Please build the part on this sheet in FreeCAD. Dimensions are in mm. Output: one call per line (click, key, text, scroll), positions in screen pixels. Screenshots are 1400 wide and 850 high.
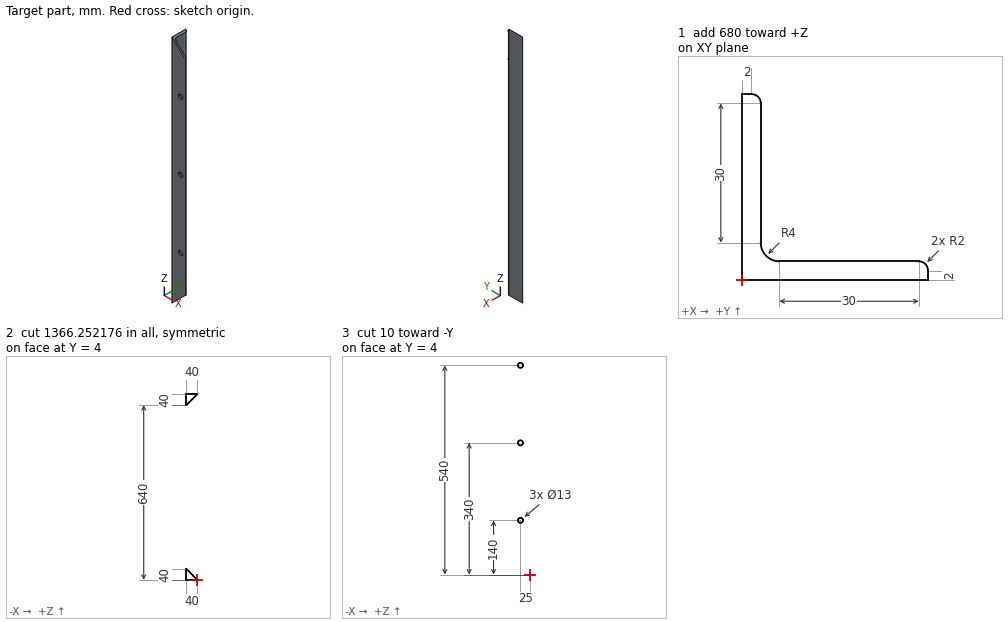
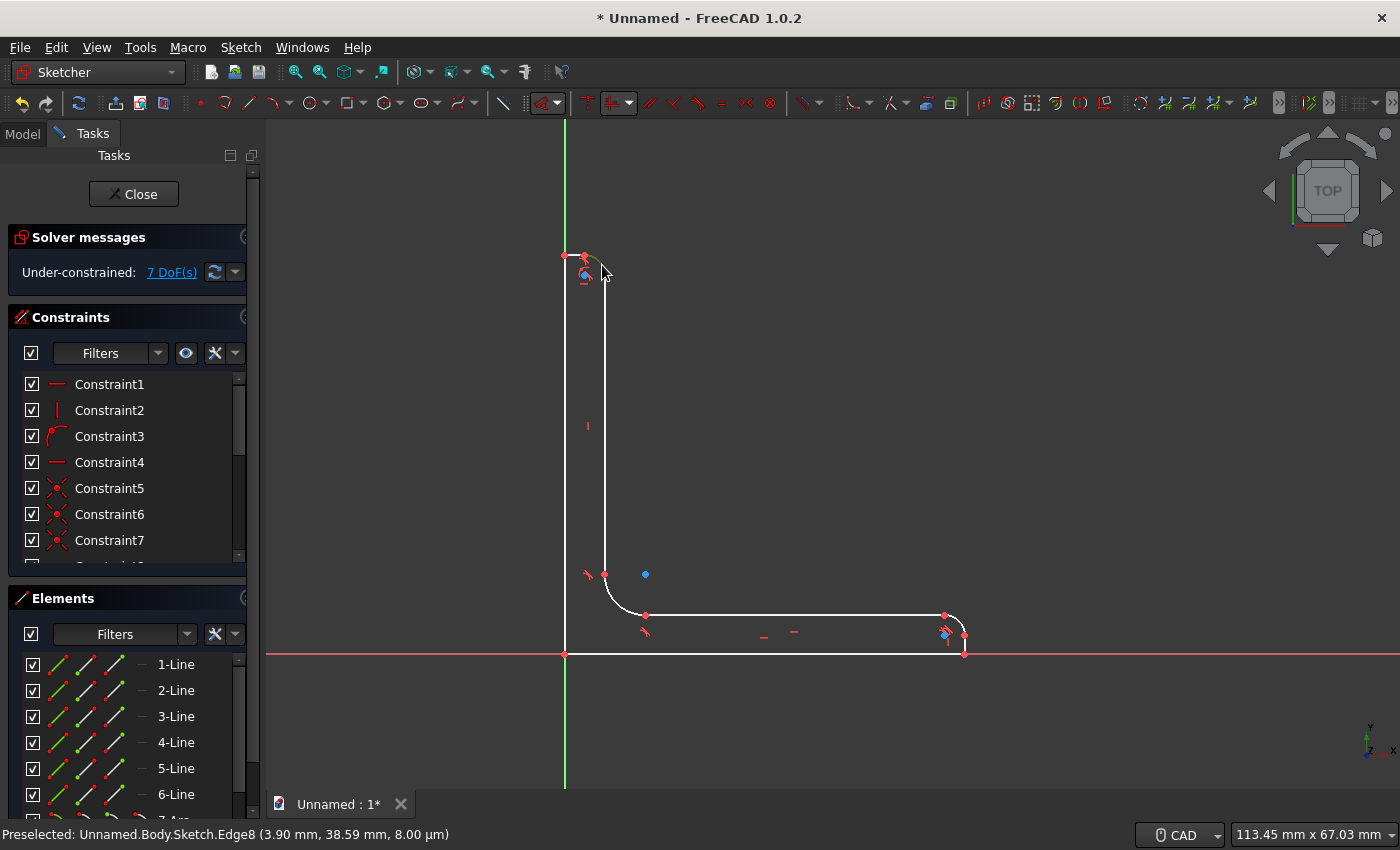
scroll(963, 626, up, 2)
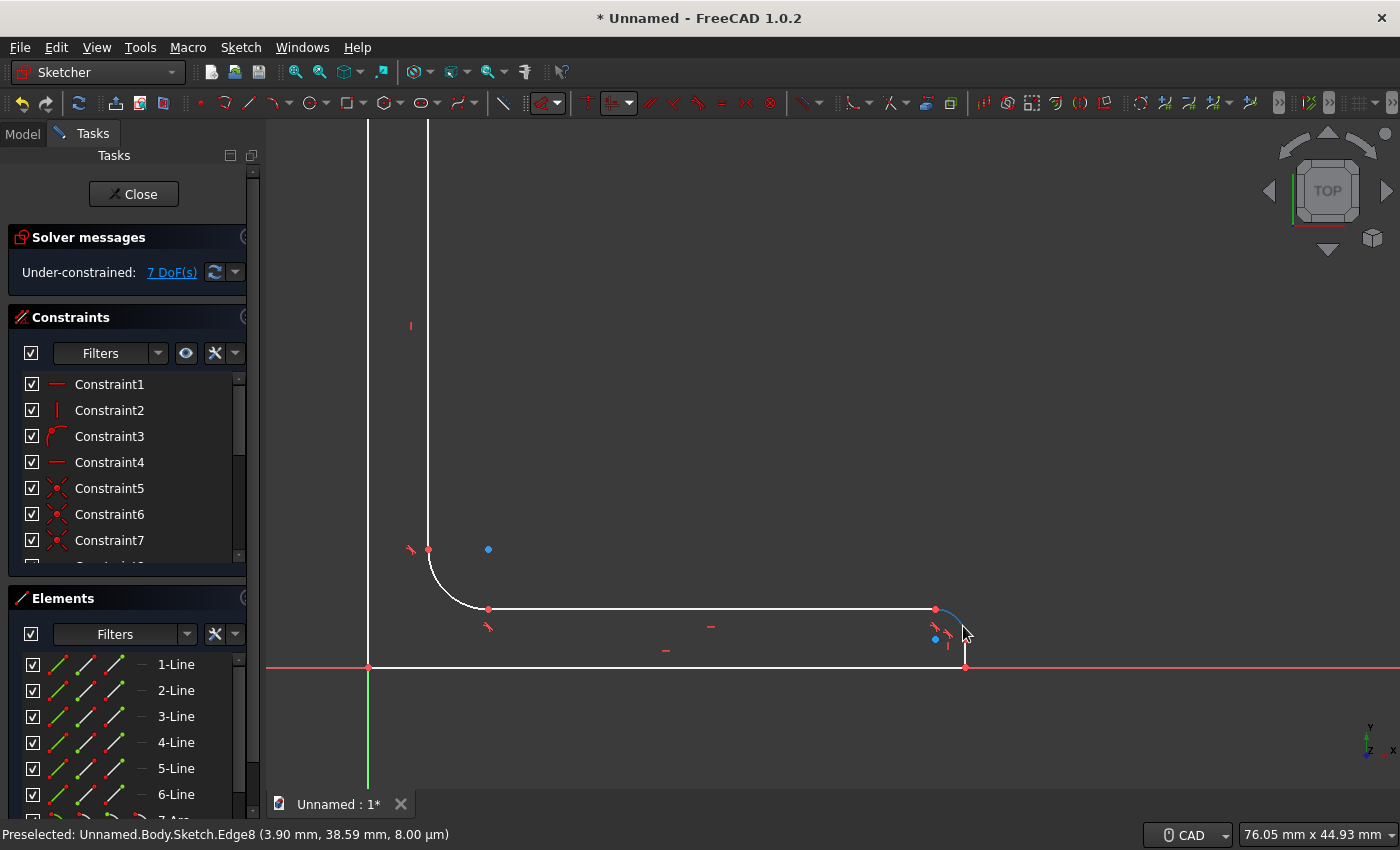
click(962, 626)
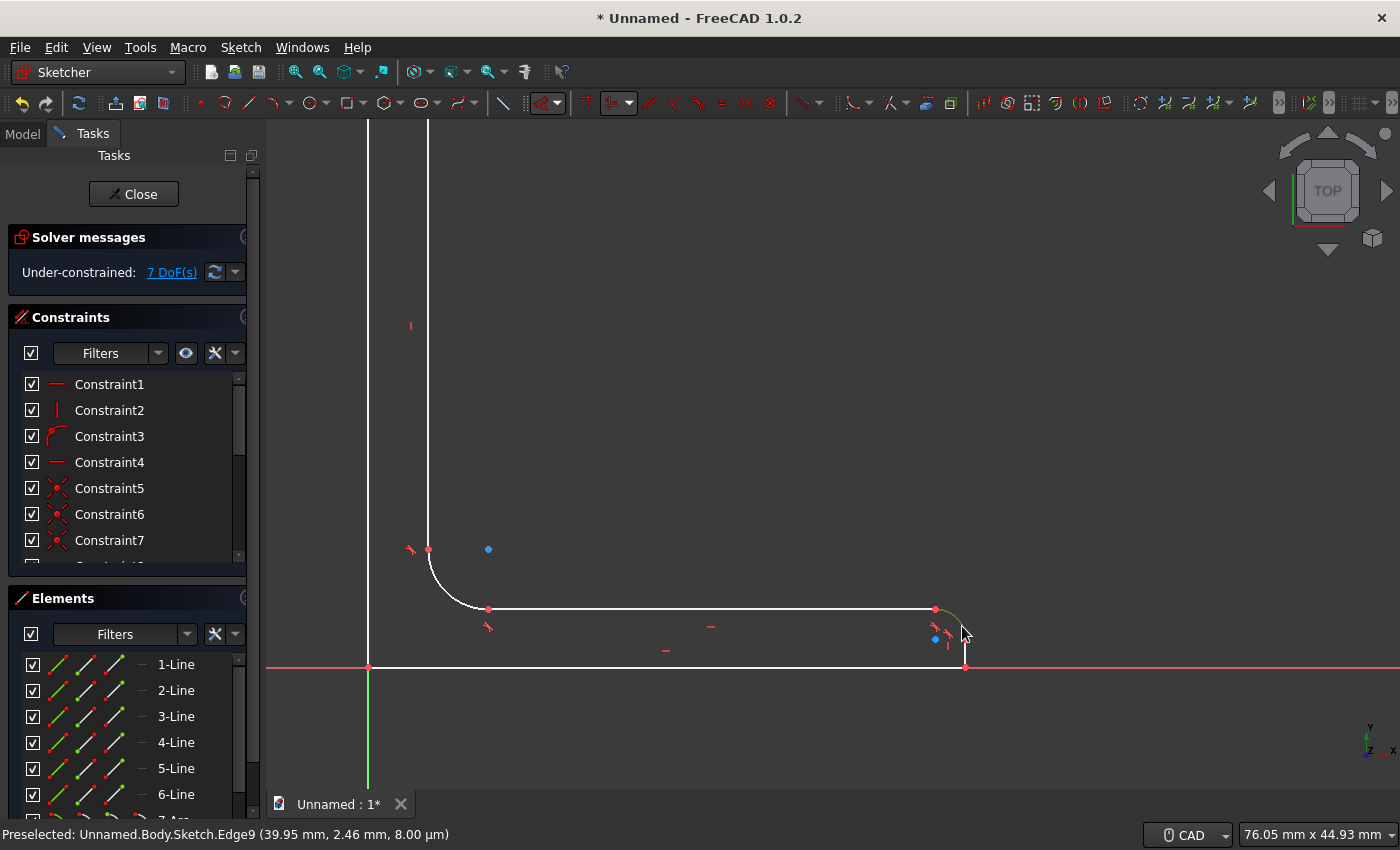
click(722, 104)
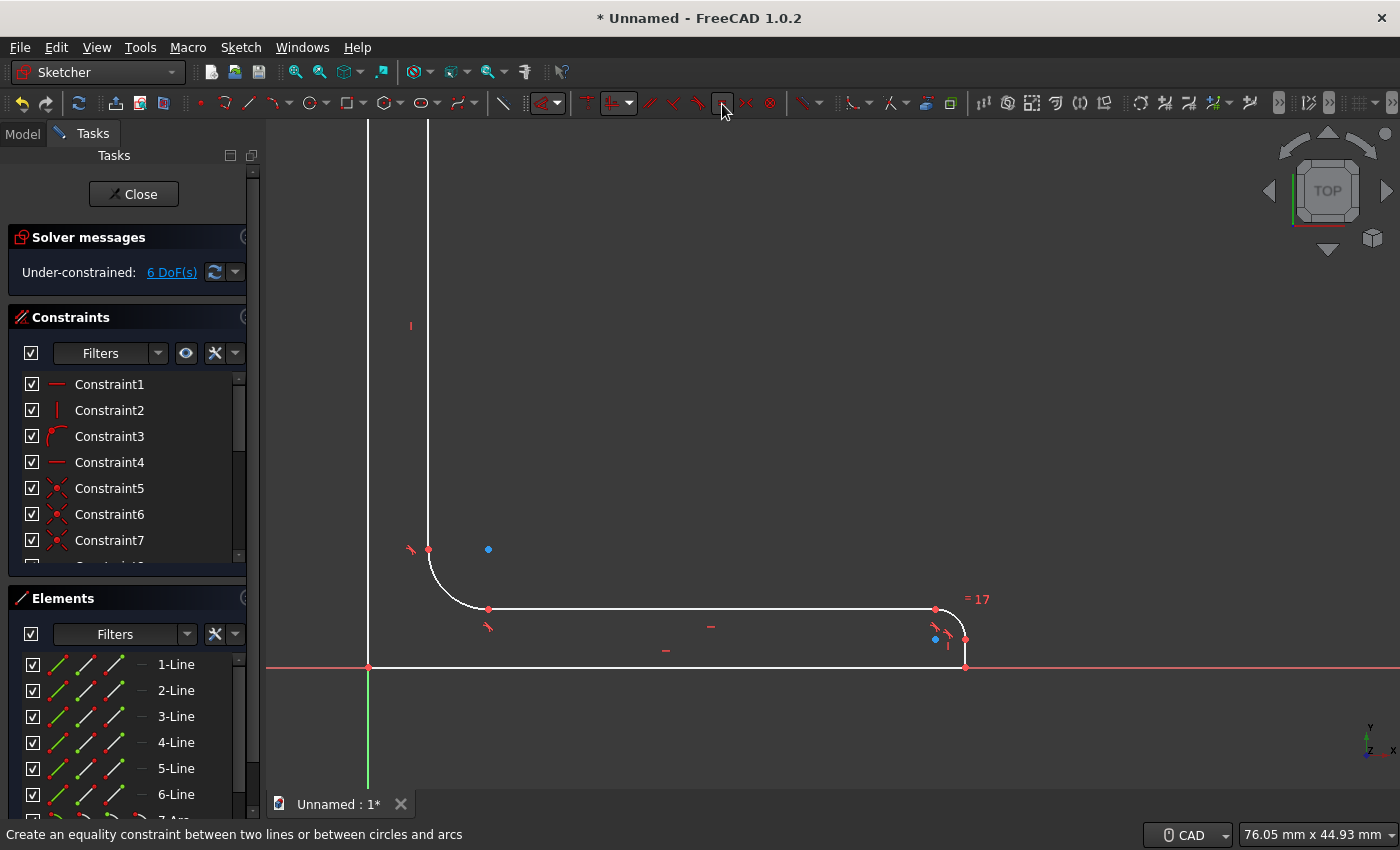
click(435, 577)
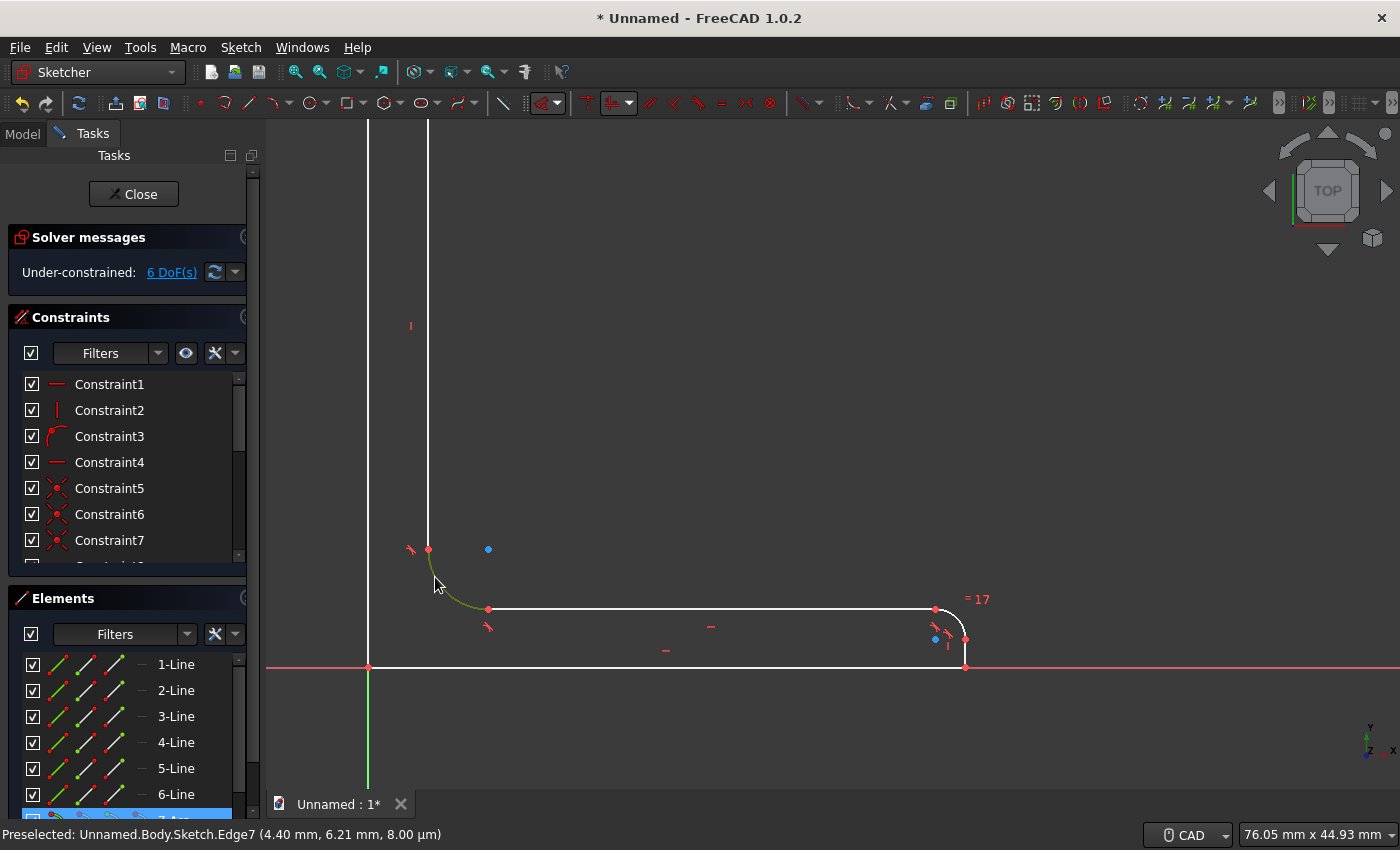
click(560, 104)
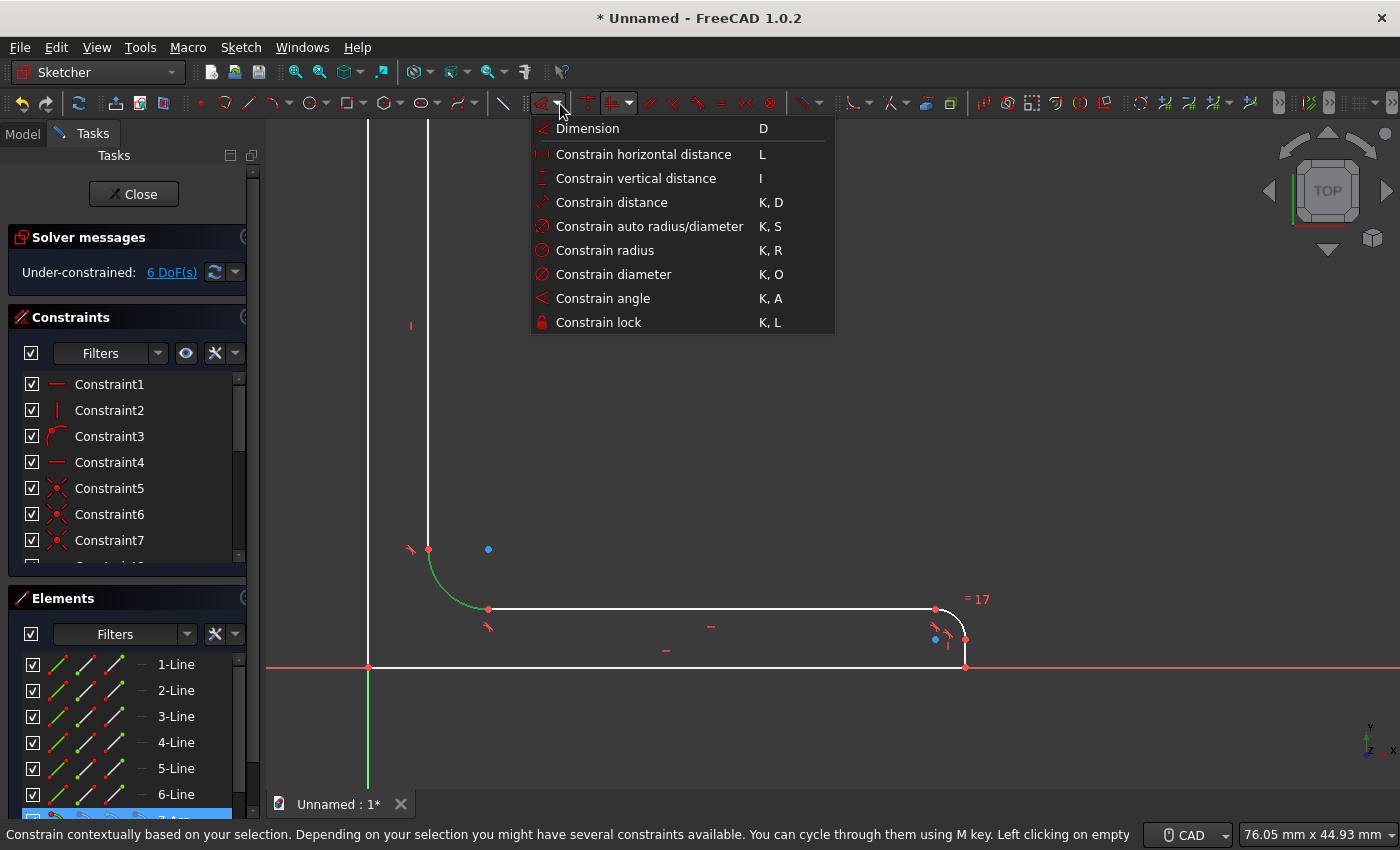
click(683, 250)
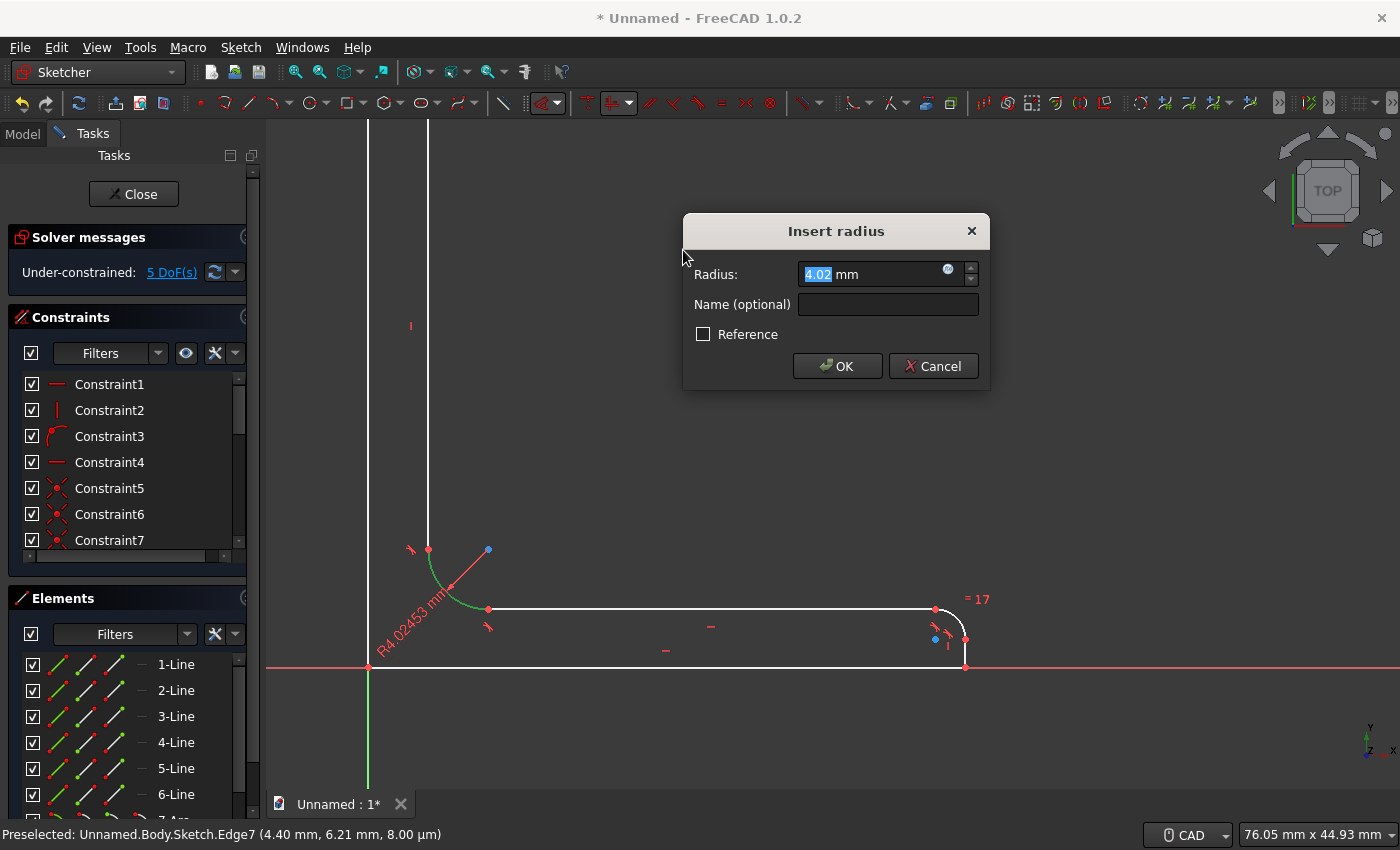
text(4)
key(Return)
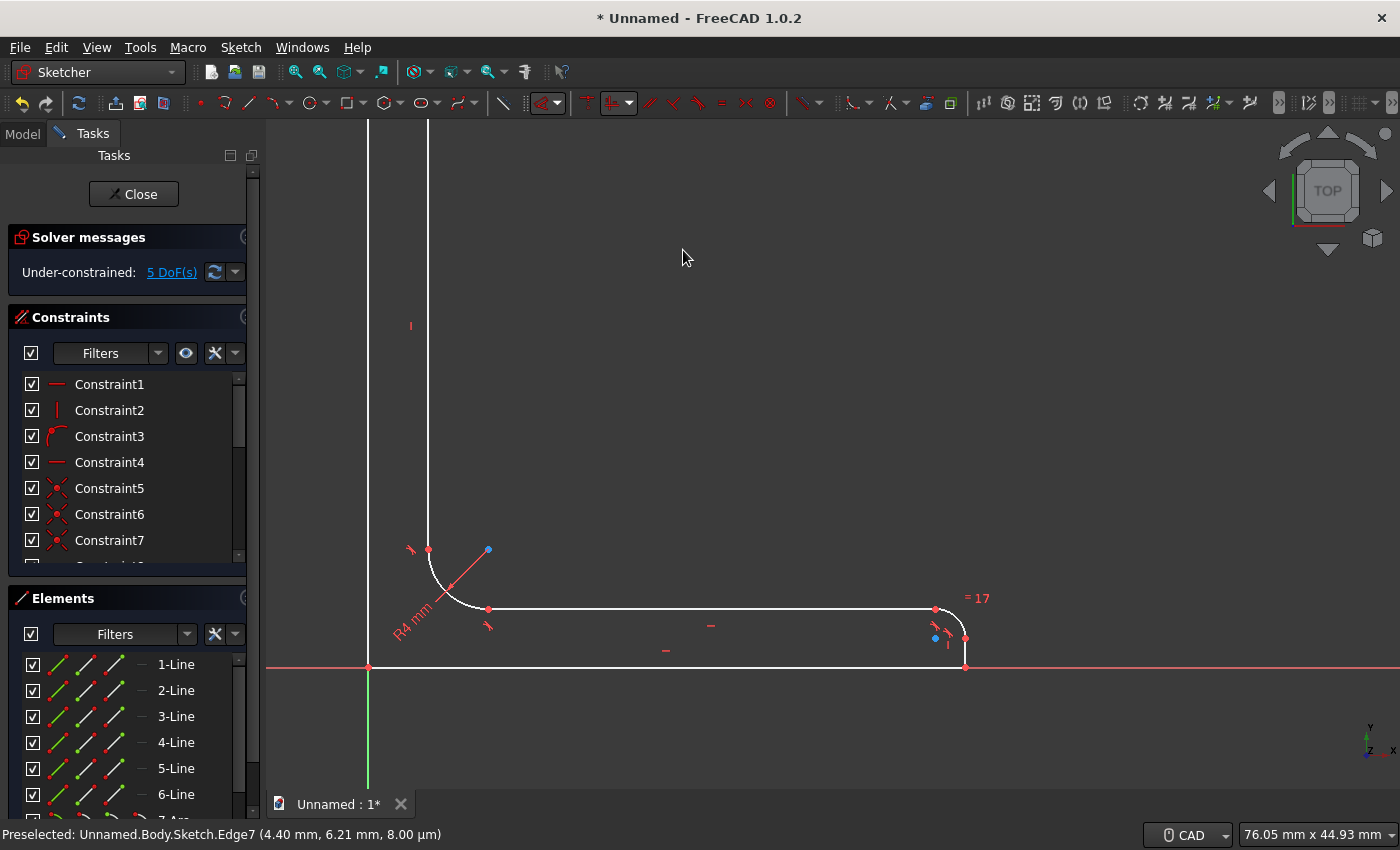
scroll(963, 626, down, 2)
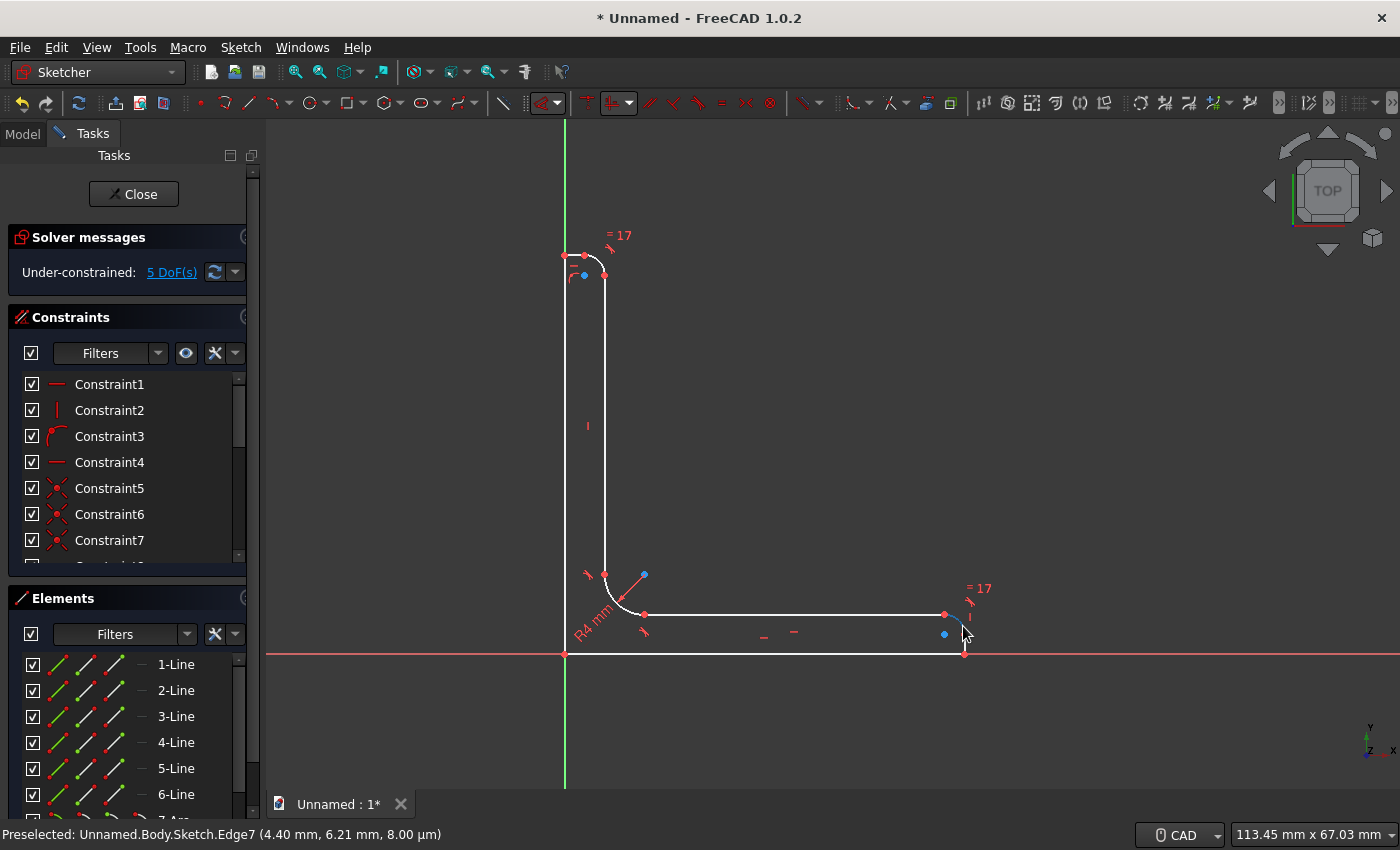
scroll(603, 266, up, 4)